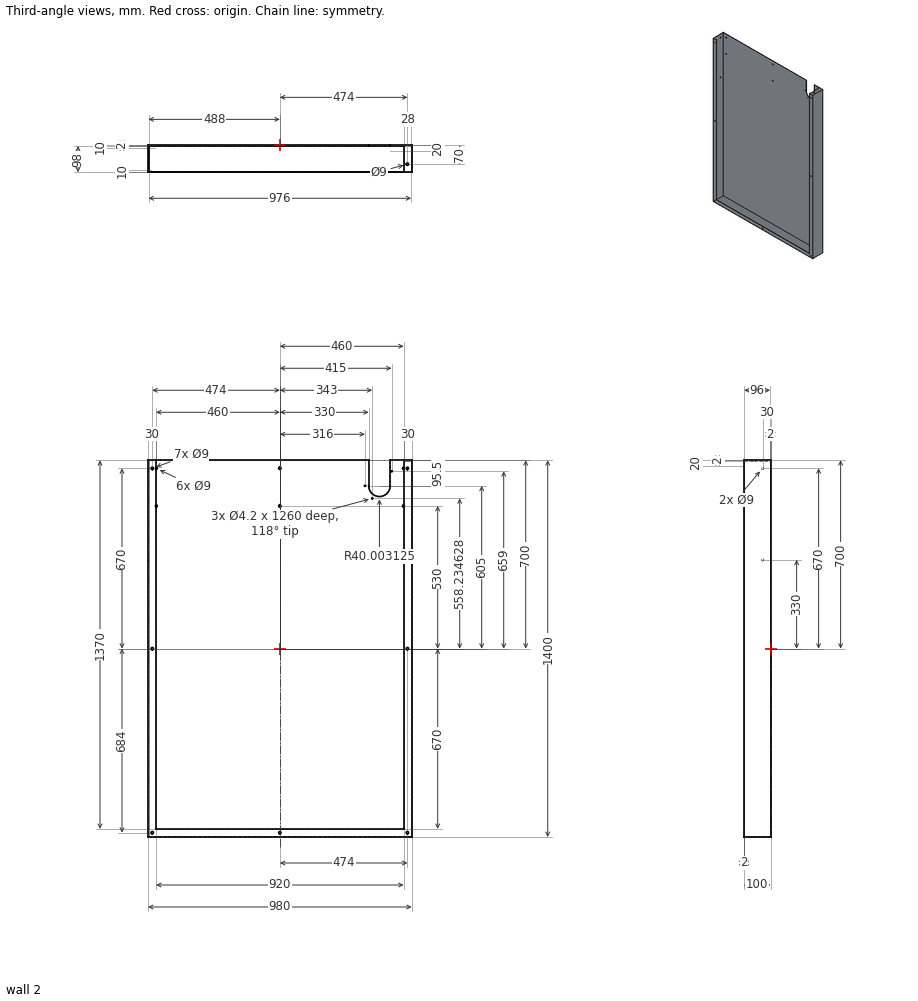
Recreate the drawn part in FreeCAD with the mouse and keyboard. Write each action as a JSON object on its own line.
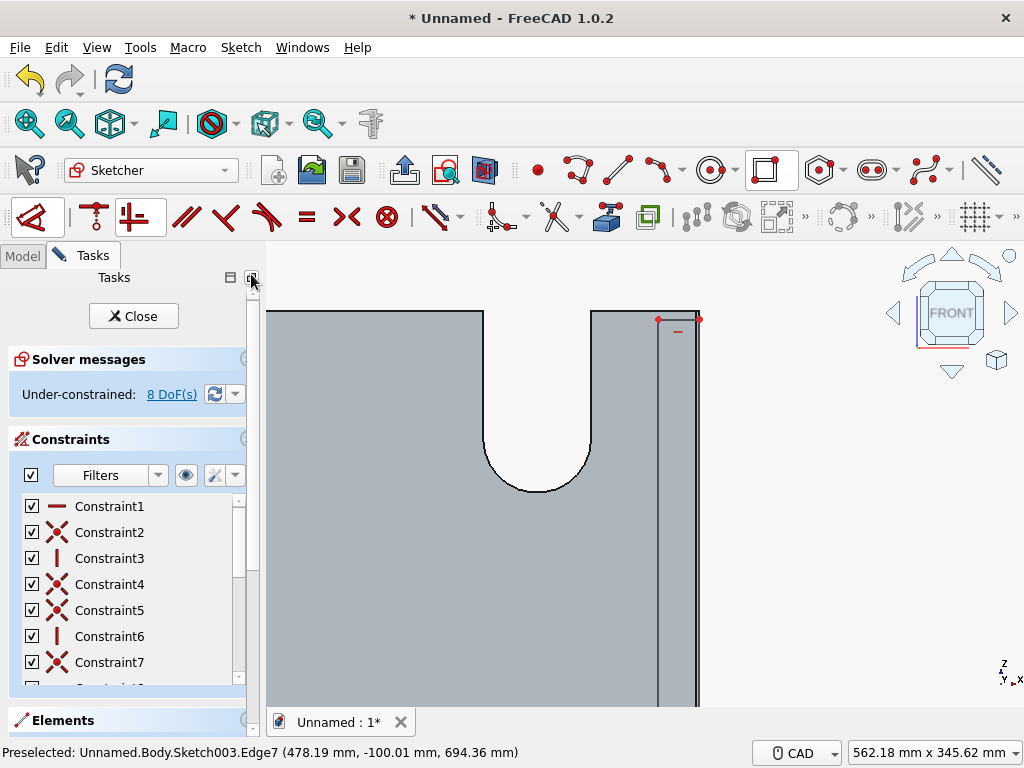
{"action": "scroll", "coordinate": [683, 319], "scroll_direction": "down", "scroll_amount": 9}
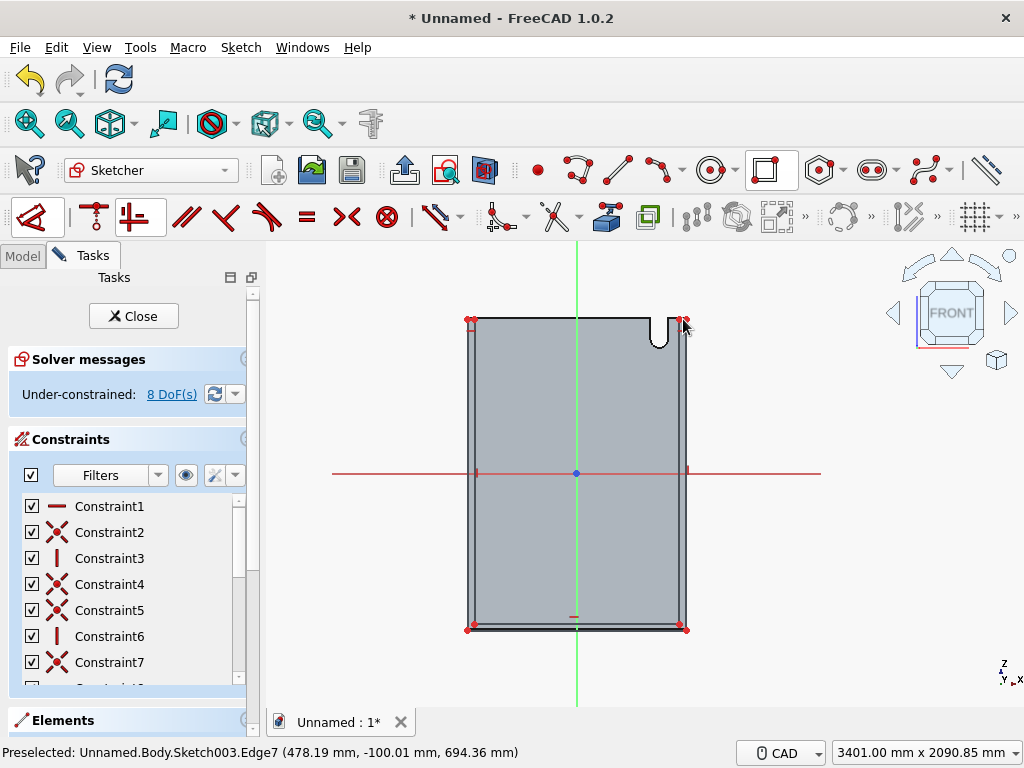
{"action": "scroll", "coordinate": [468, 319], "scroll_direction": "up", "scroll_amount": 3}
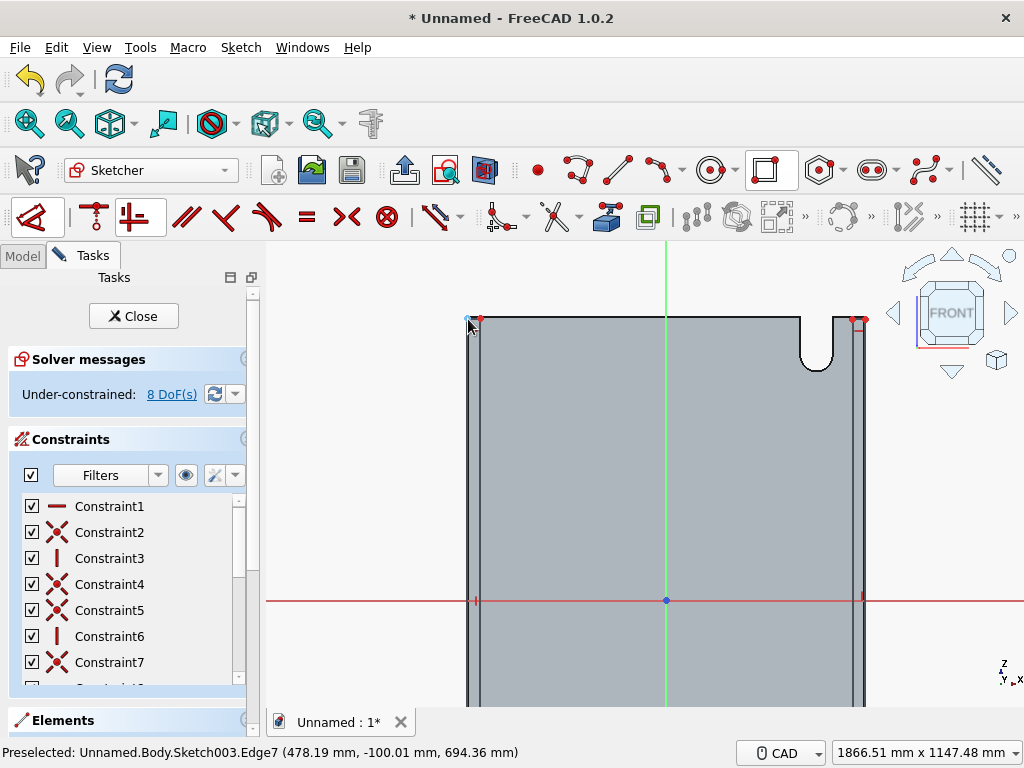
{"action": "left_click", "coordinate": [467, 319]}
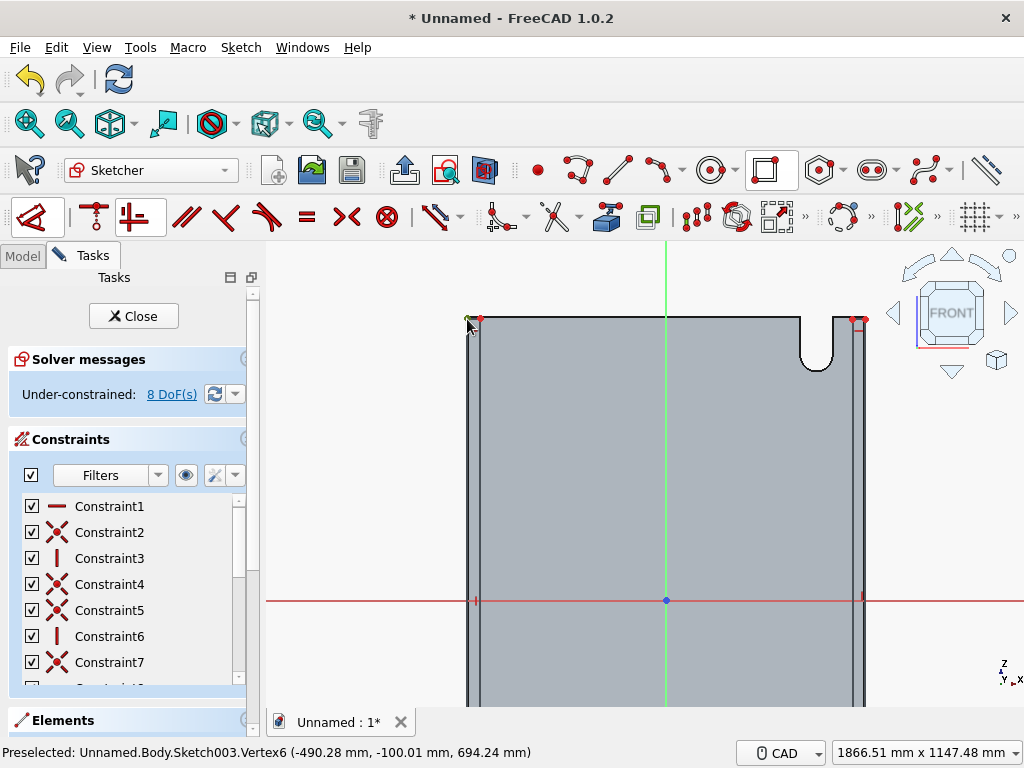
{"action": "scroll", "coordinate": [467, 320], "scroll_direction": "down", "scroll_amount": 3}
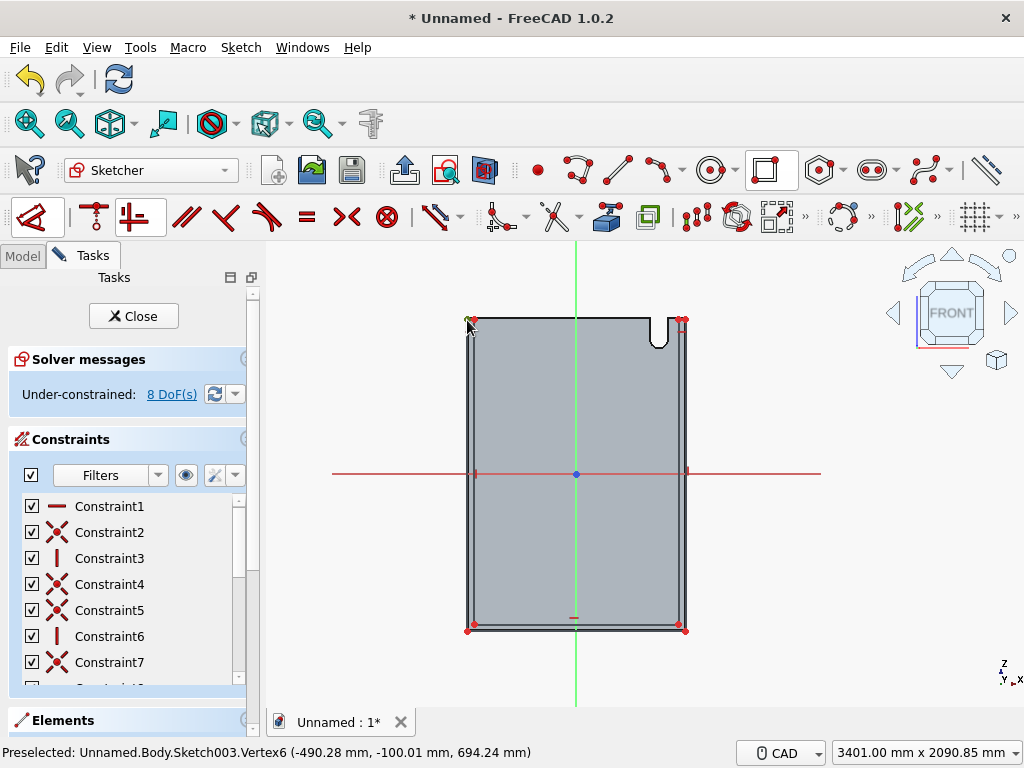
{"action": "scroll", "coordinate": [686, 320], "scroll_direction": "up", "scroll_amount": 3}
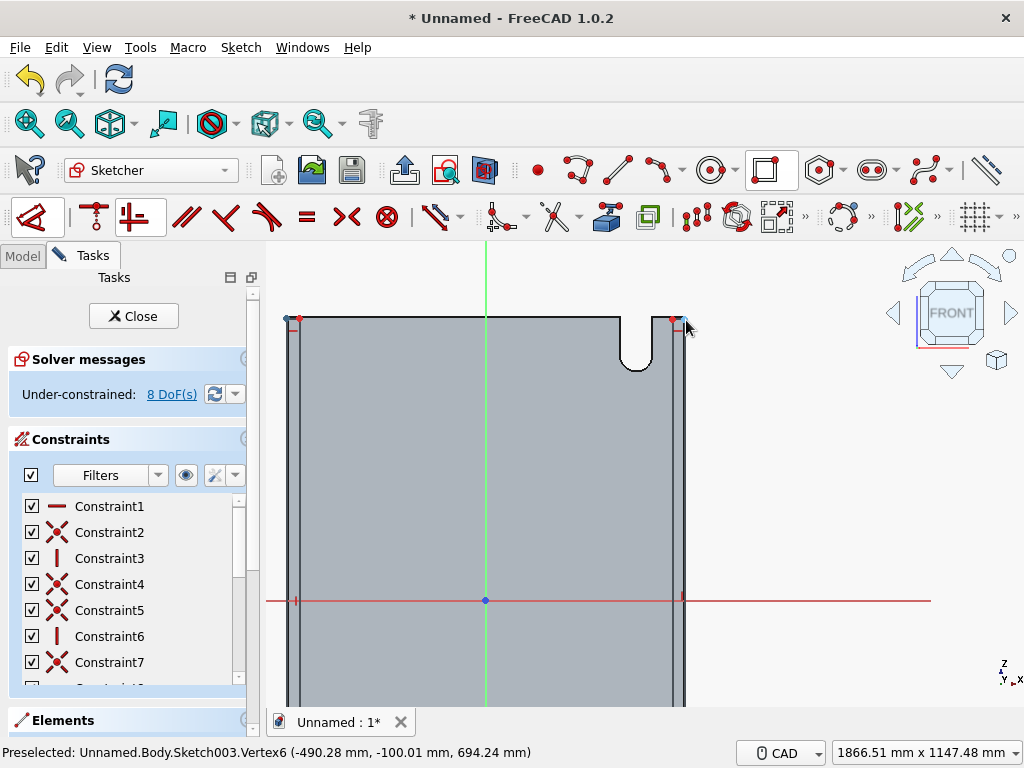
{"action": "left_click", "coordinate": [685, 319]}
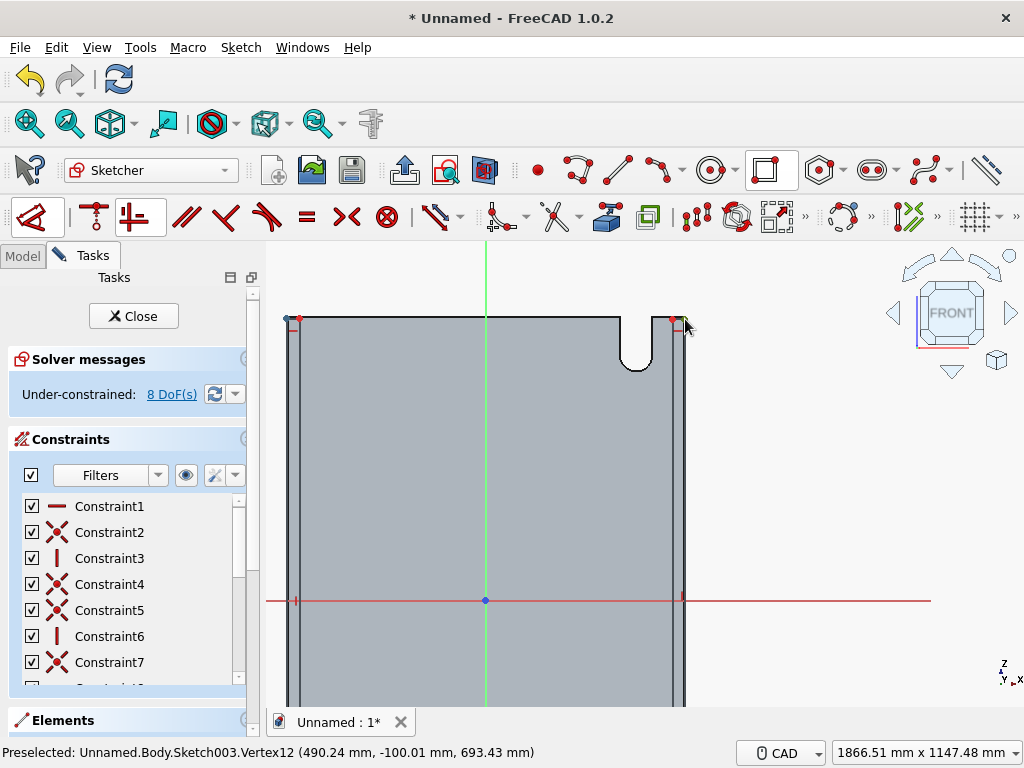
{"action": "left_click", "coordinate": [486, 650]}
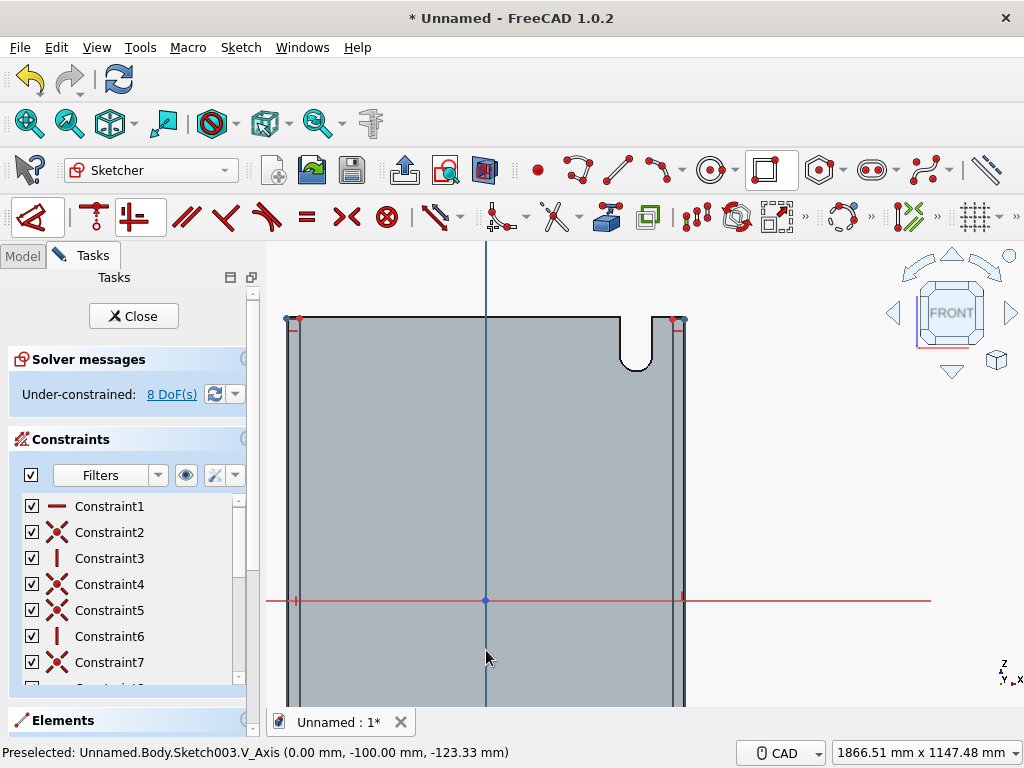
{"action": "left_click", "coordinate": [348, 218]}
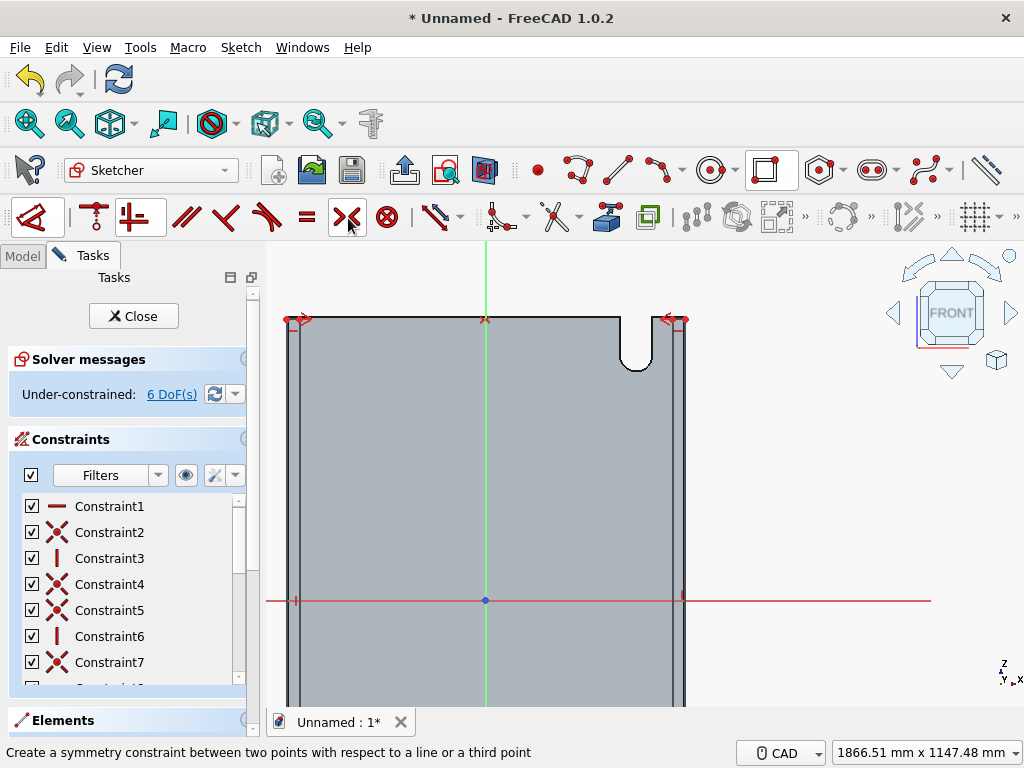
{"action": "scroll", "coordinate": [687, 320], "scroll_direction": "down", "scroll_amount": 3}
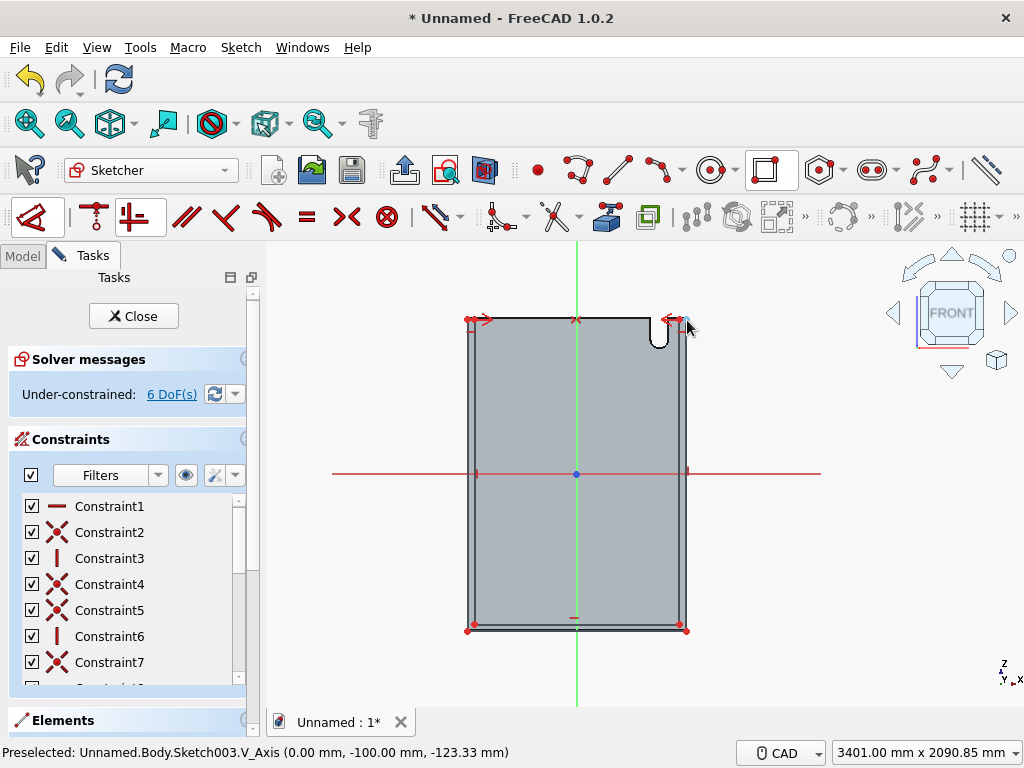
{"action": "scroll", "coordinate": [471, 320], "scroll_direction": "up", "scroll_amount": 9}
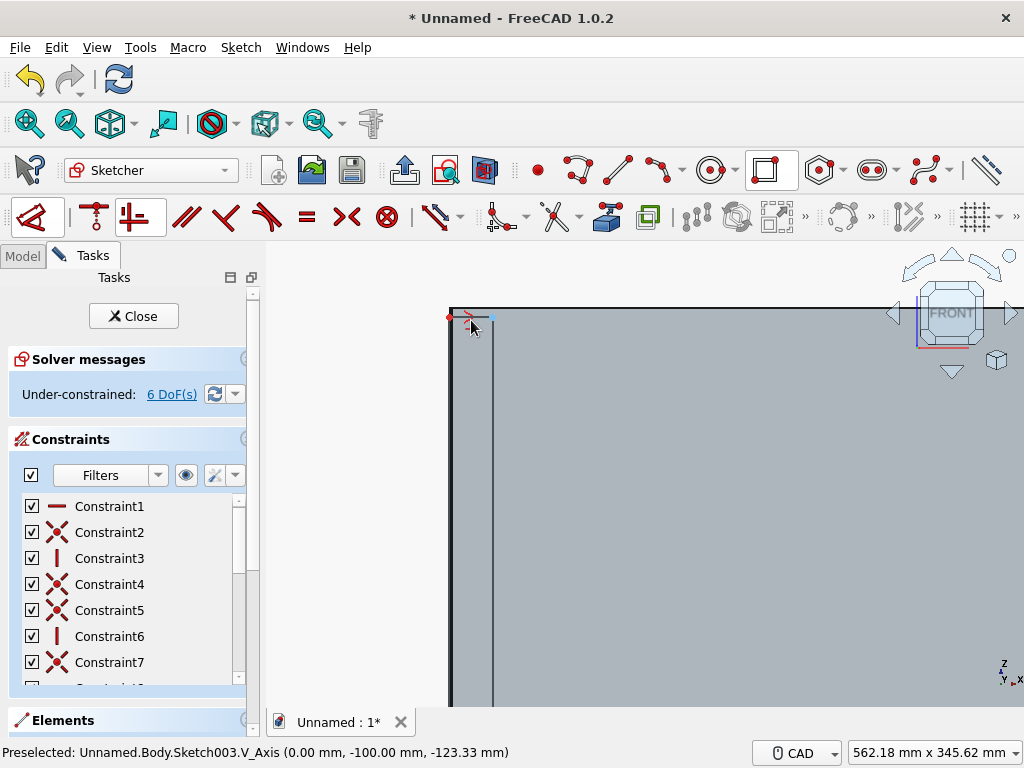
{"action": "left_click", "coordinate": [467, 317]}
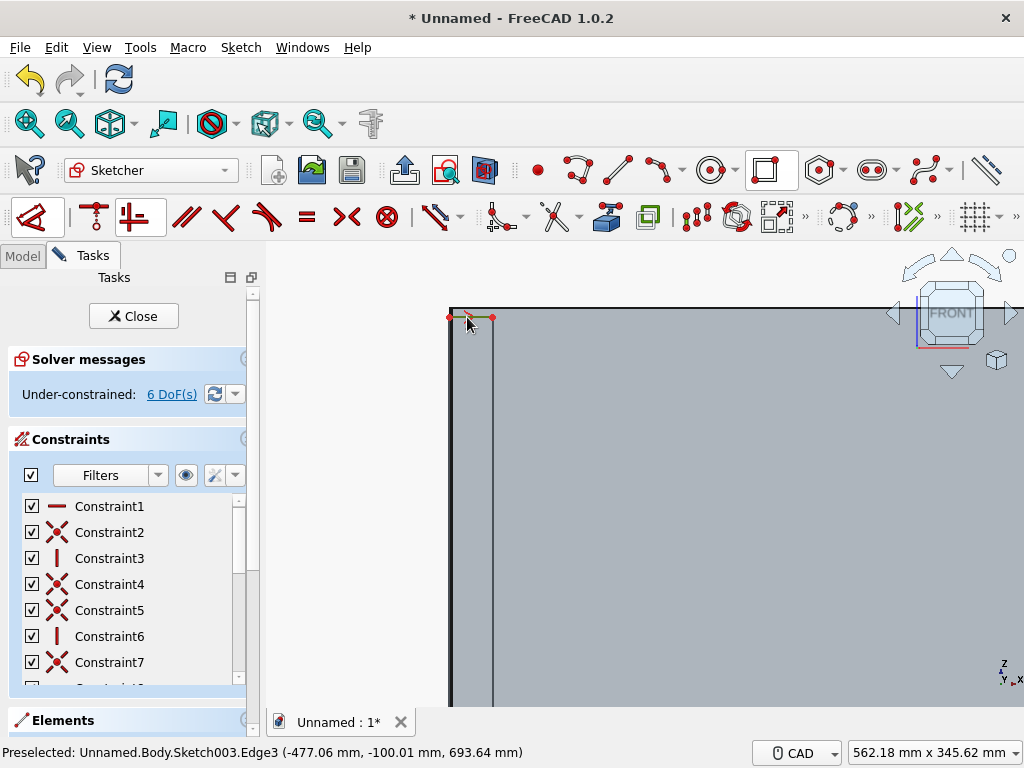
{"action": "left_click", "coordinate": [58, 218]}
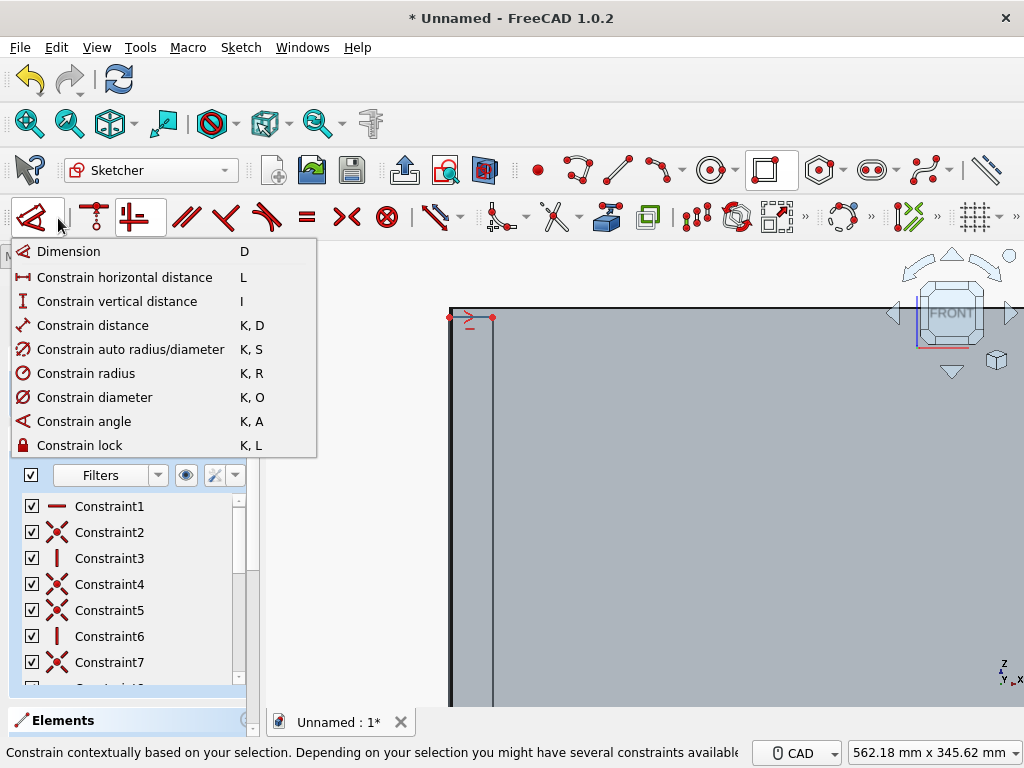
{"action": "left_click", "coordinate": [164, 277]}